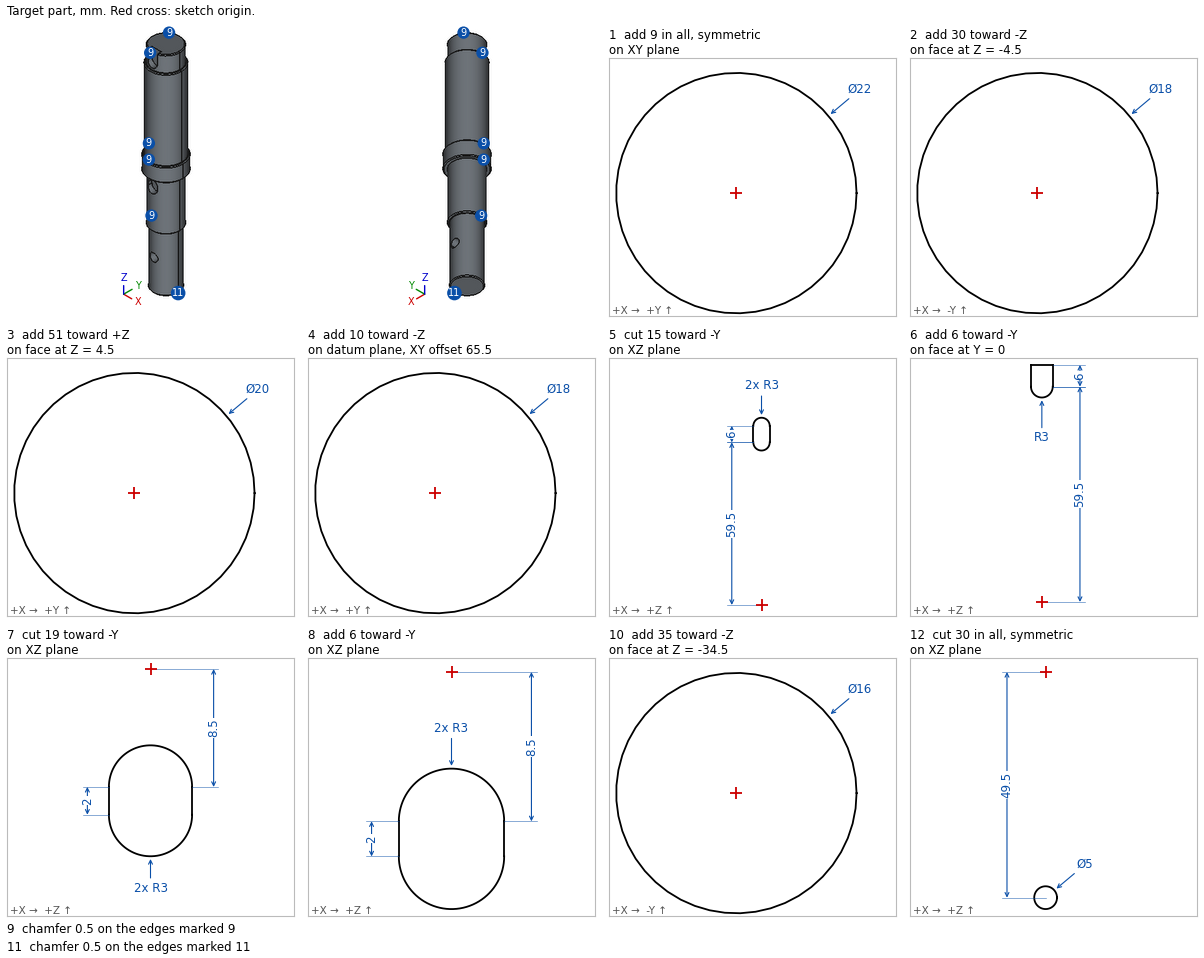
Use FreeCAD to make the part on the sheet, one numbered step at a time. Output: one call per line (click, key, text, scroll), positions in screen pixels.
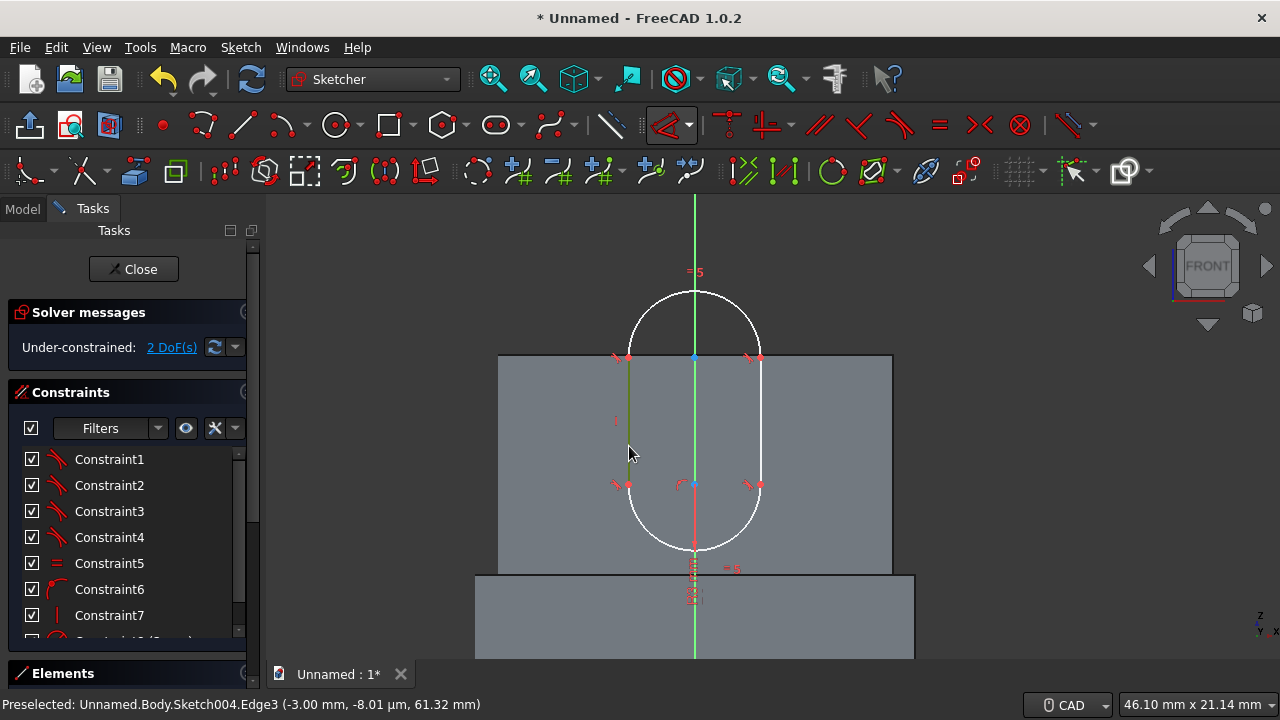
click(692, 126)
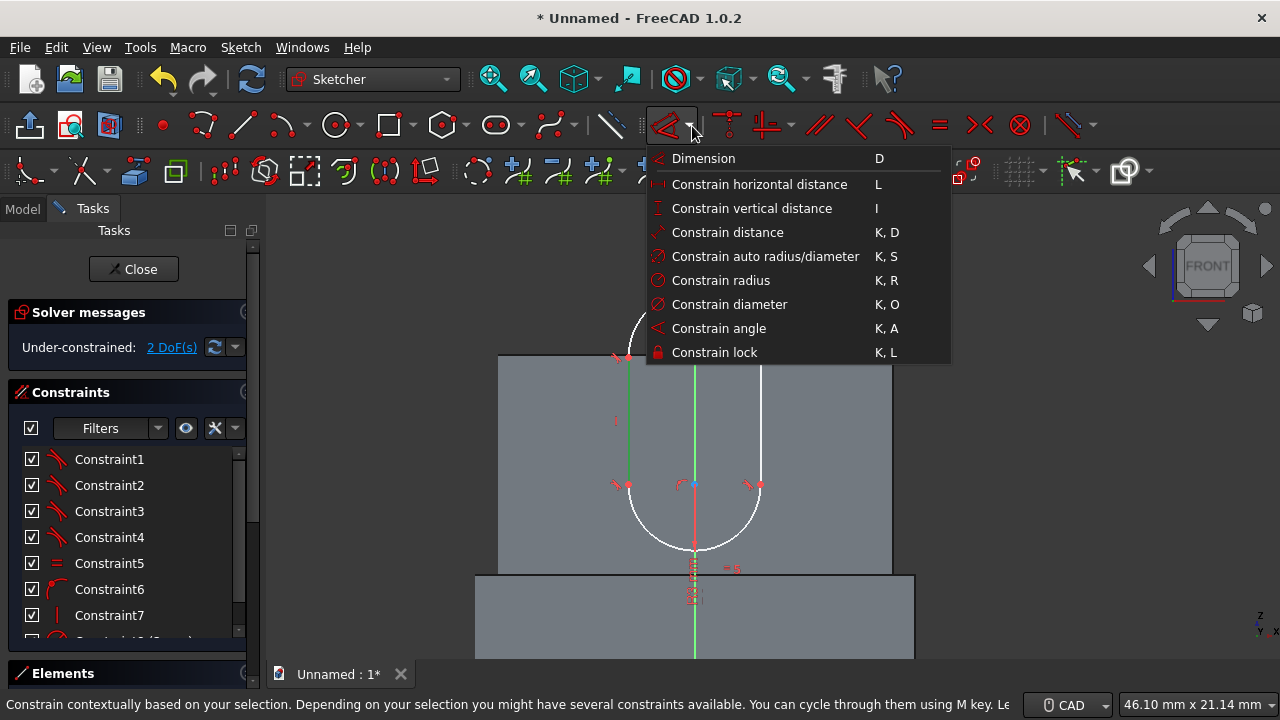
click(799, 208)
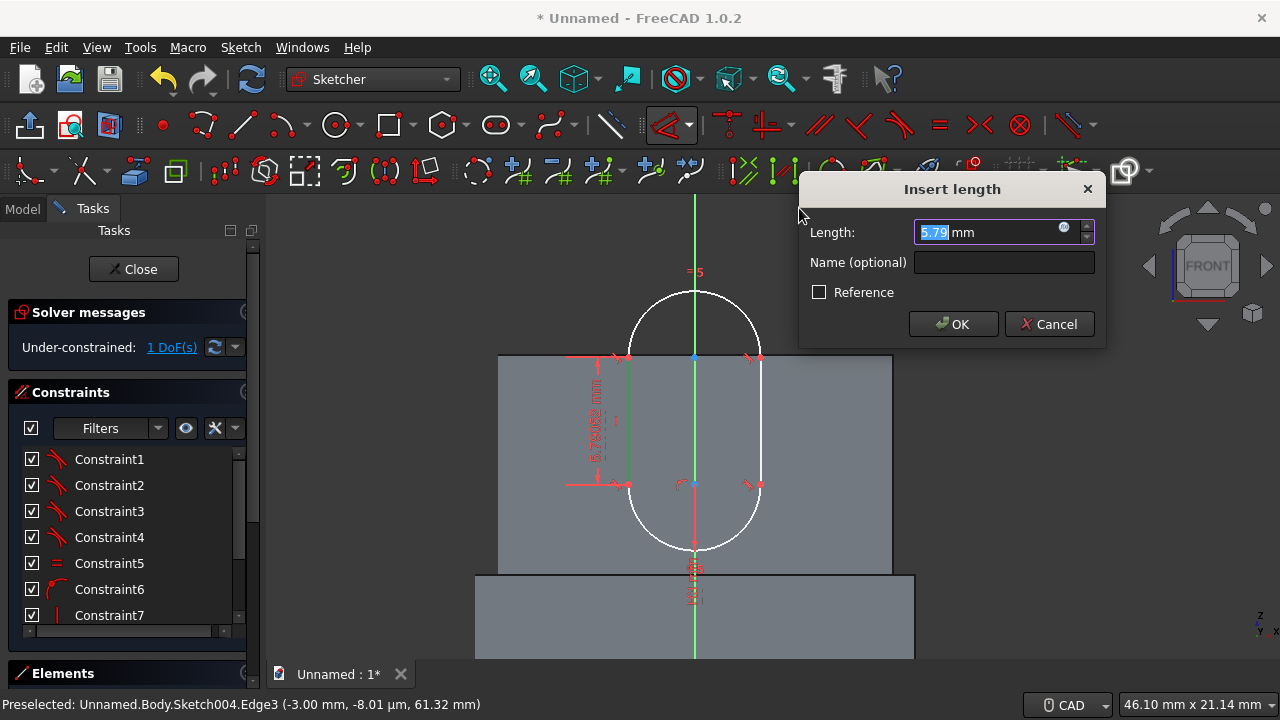
text(6)
key(Return)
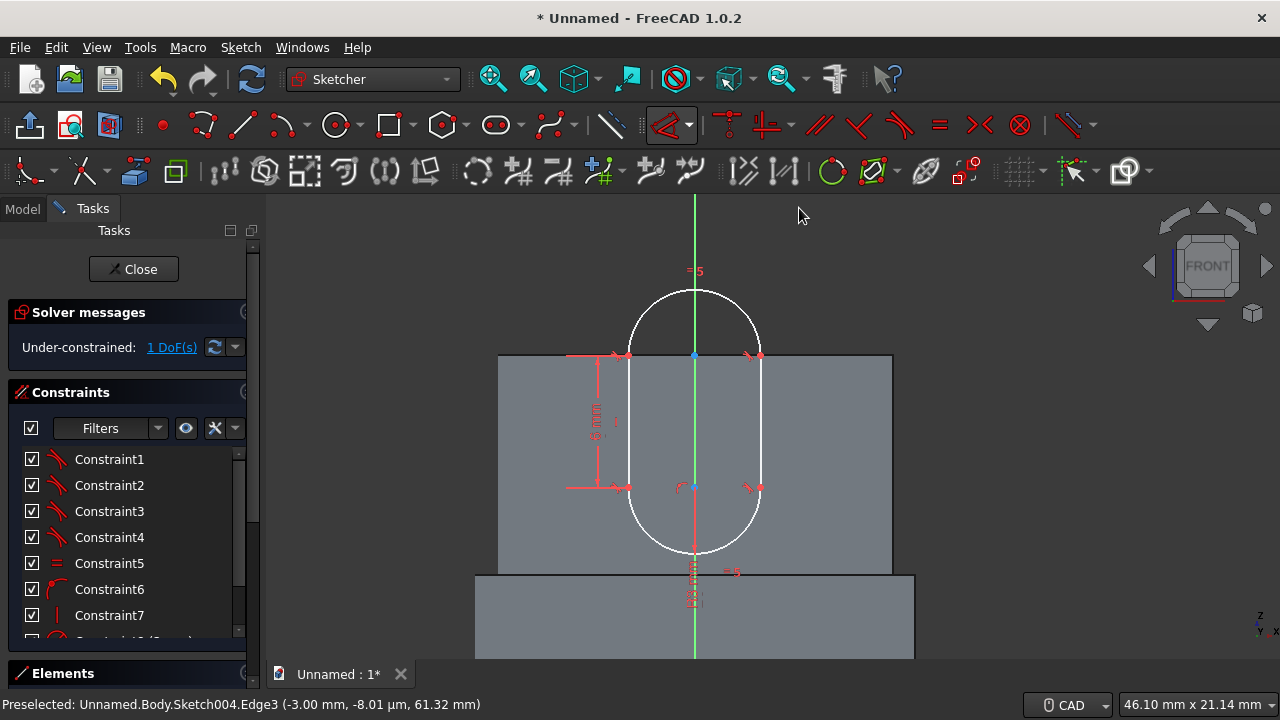
click(629, 488)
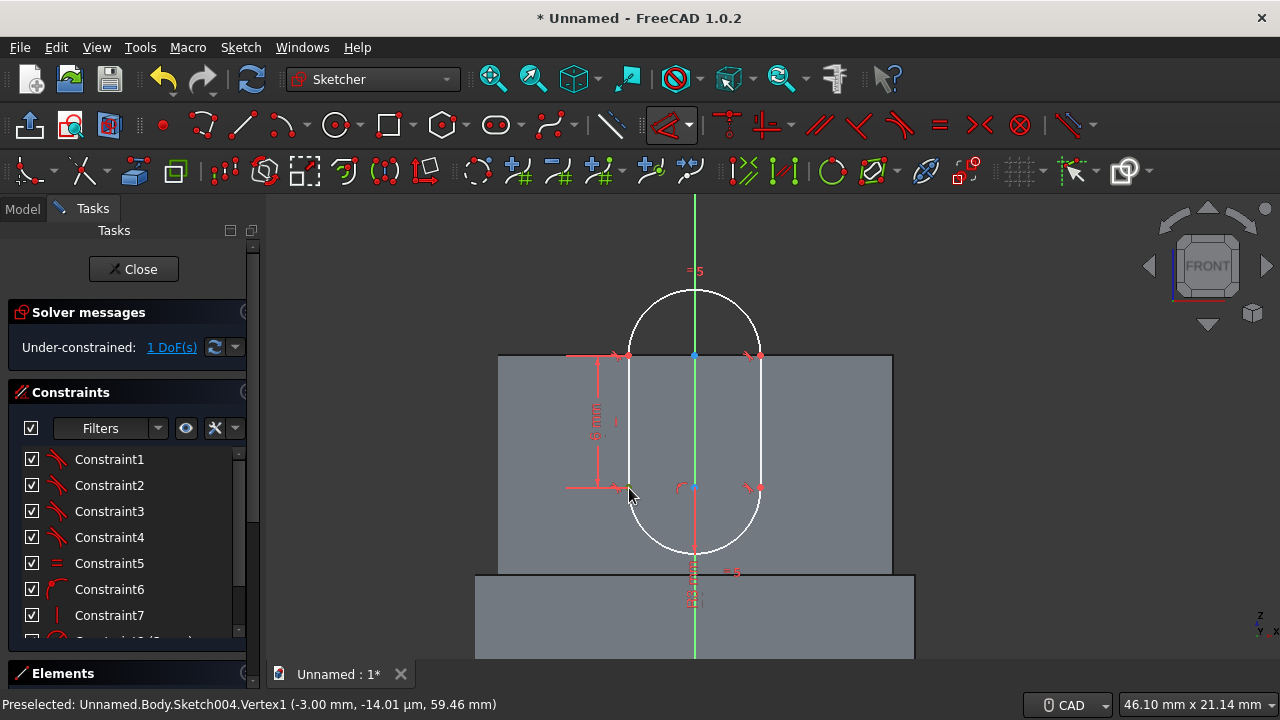
click(692, 126)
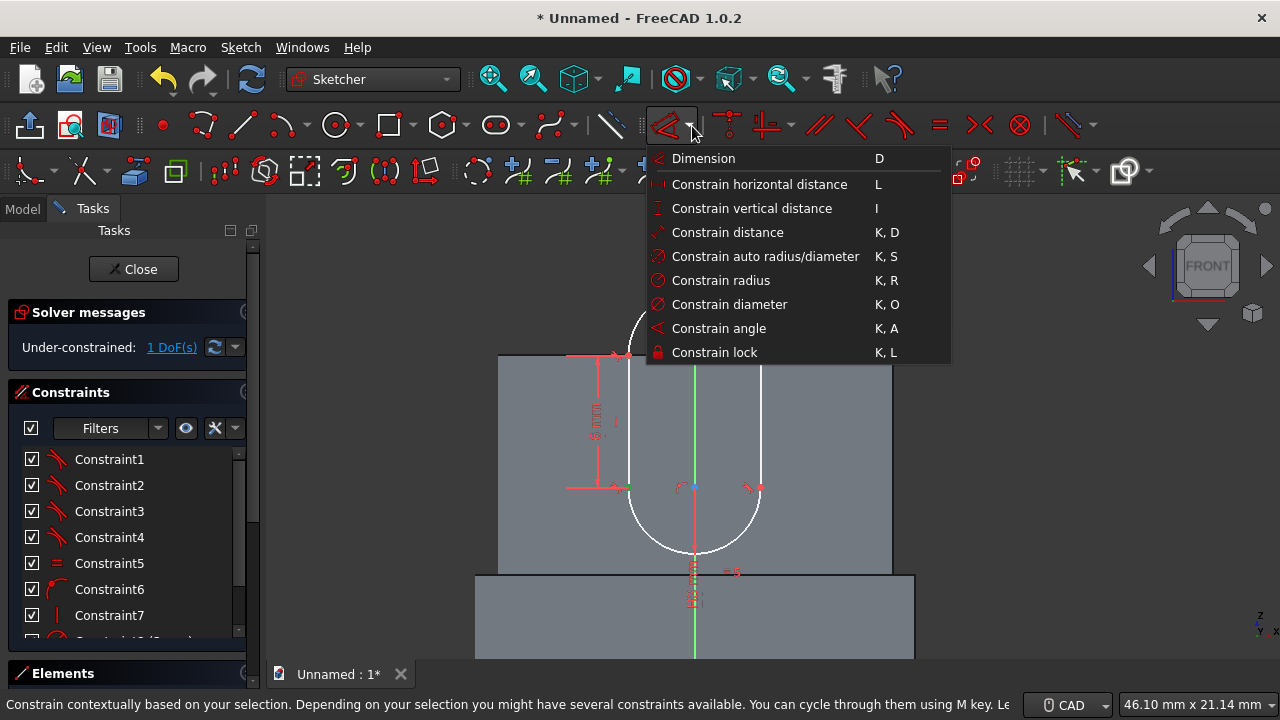
click(799, 208)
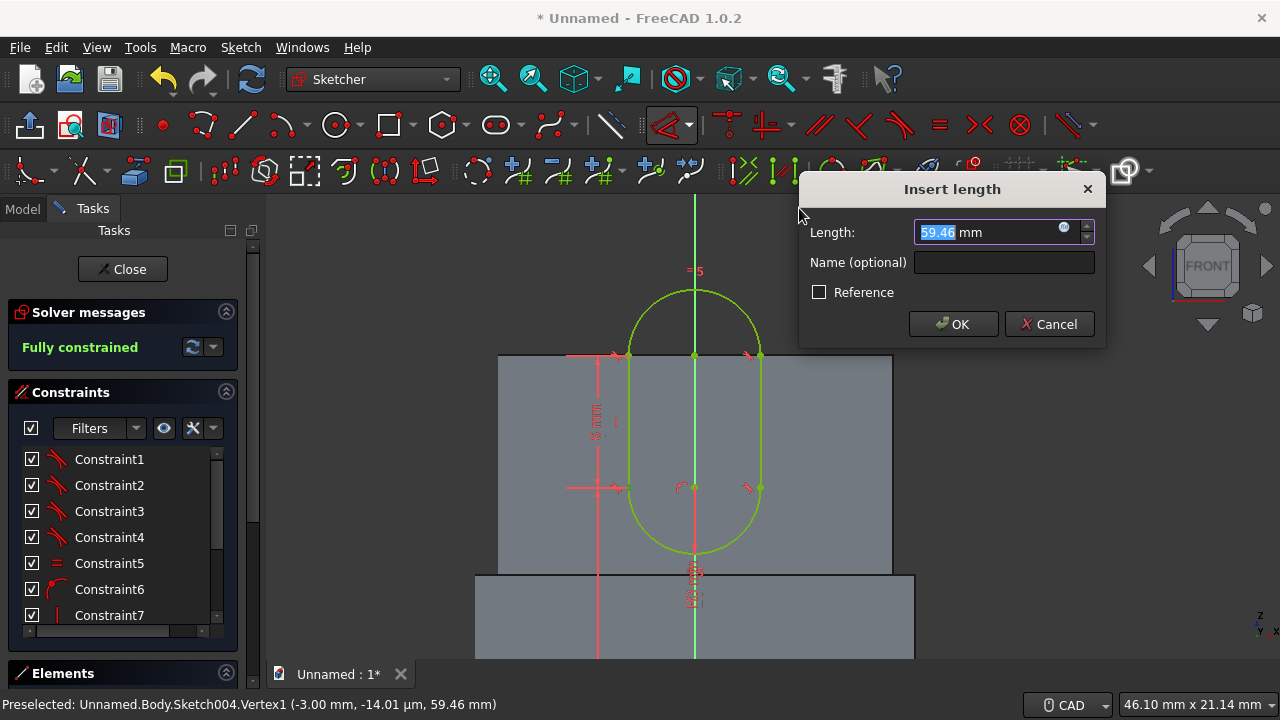
text(59.5)
key(Return)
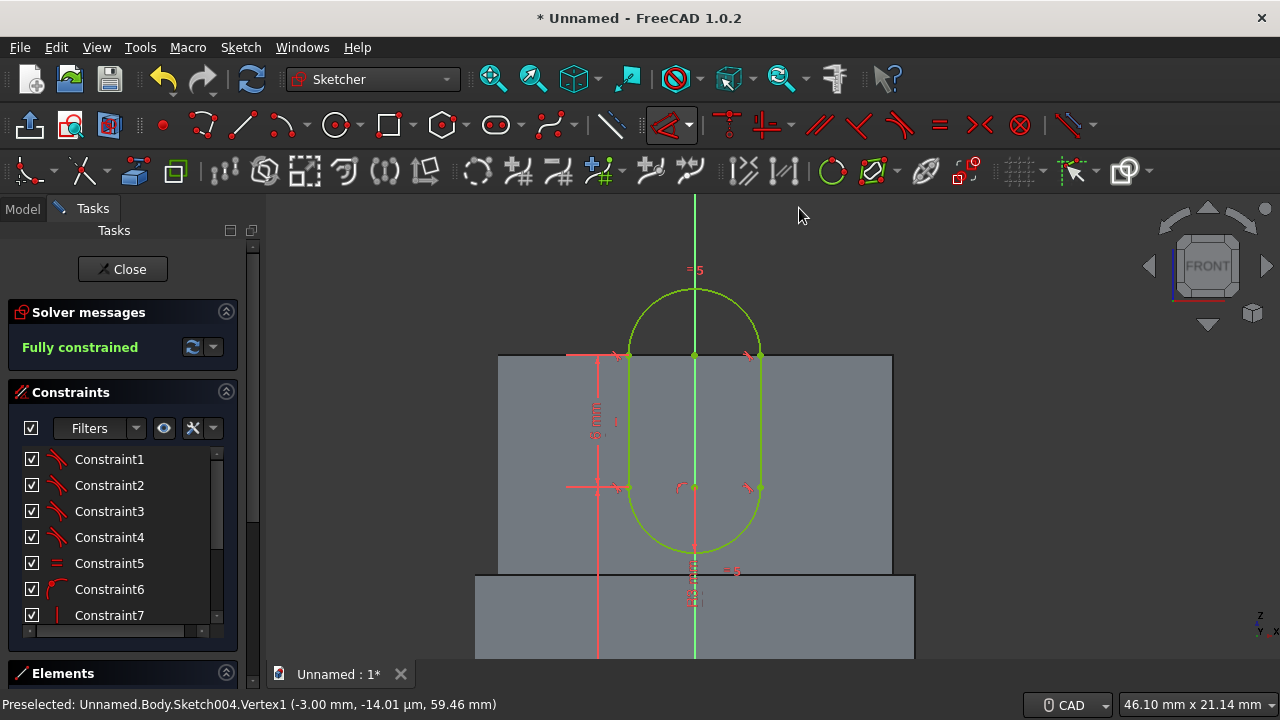
click(123, 269)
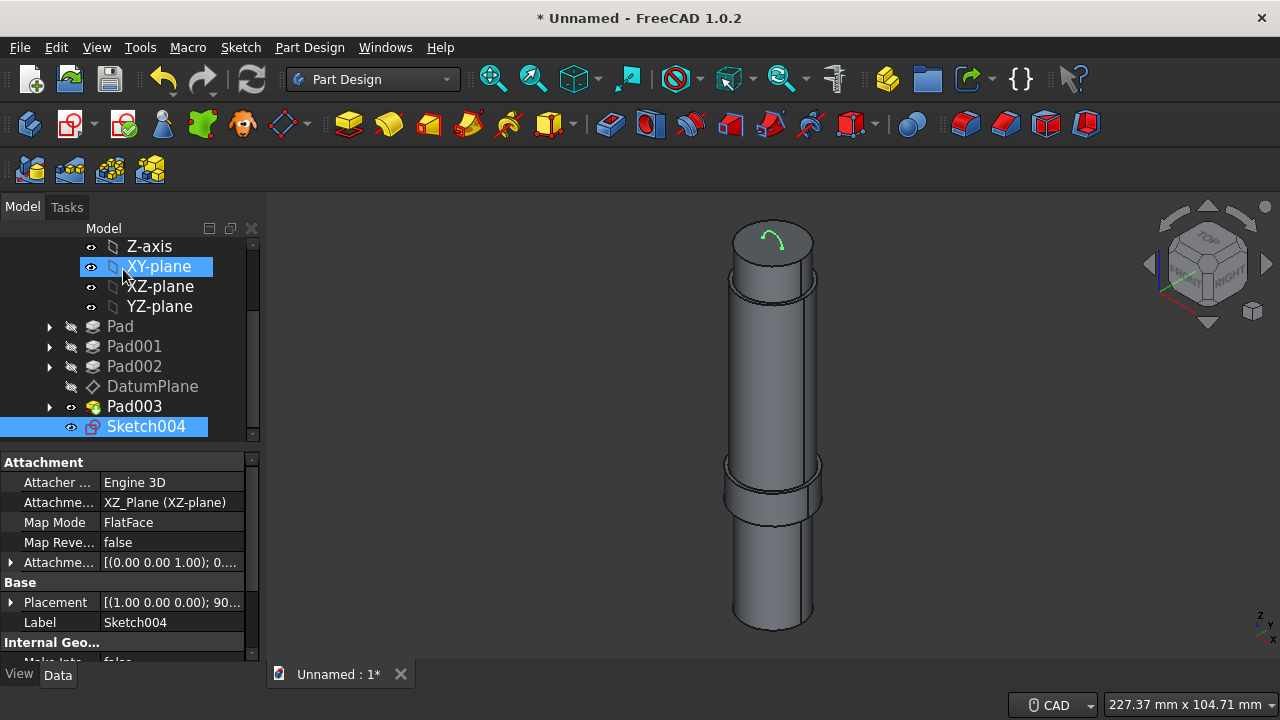
click(612, 124)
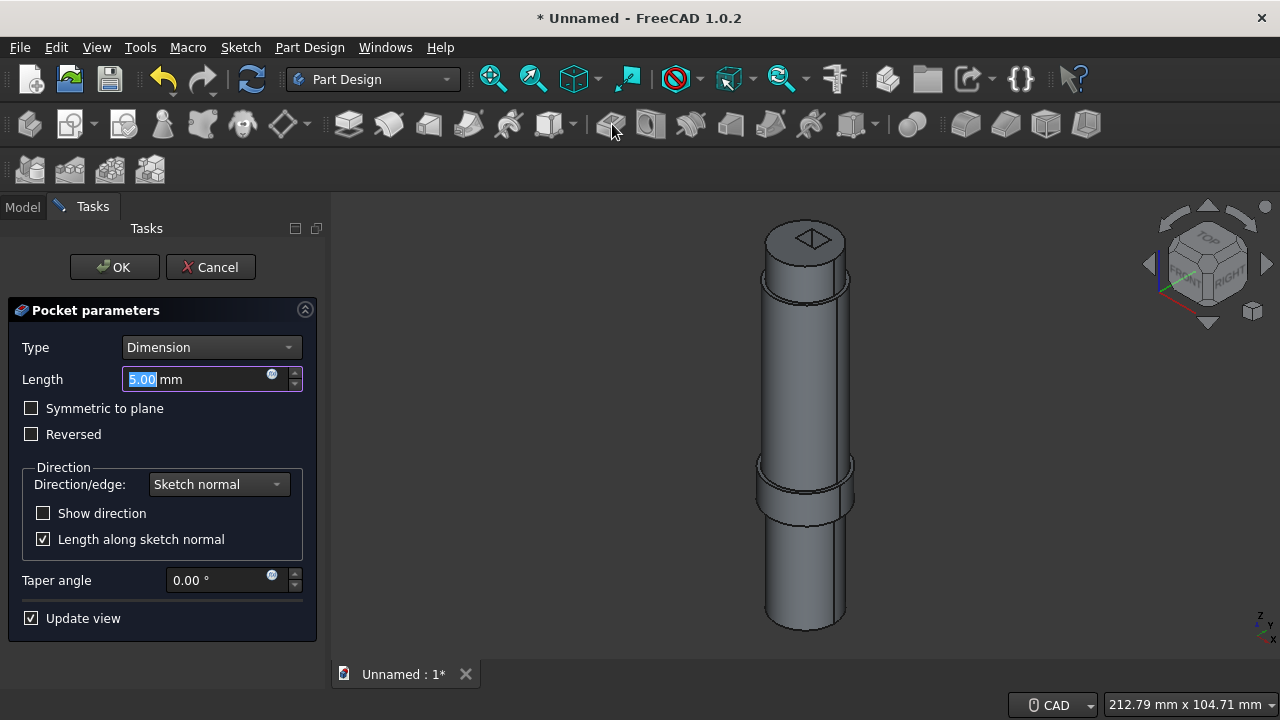
text(15)
key(Tab)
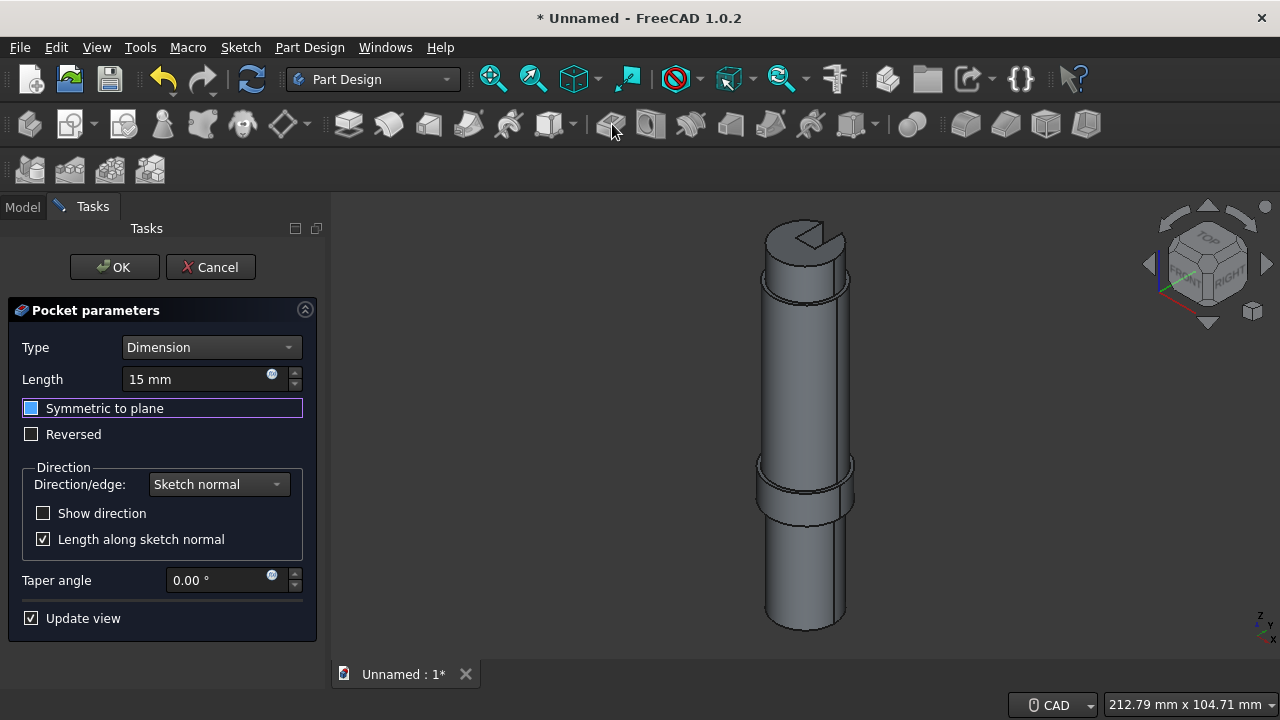
click(30, 434)